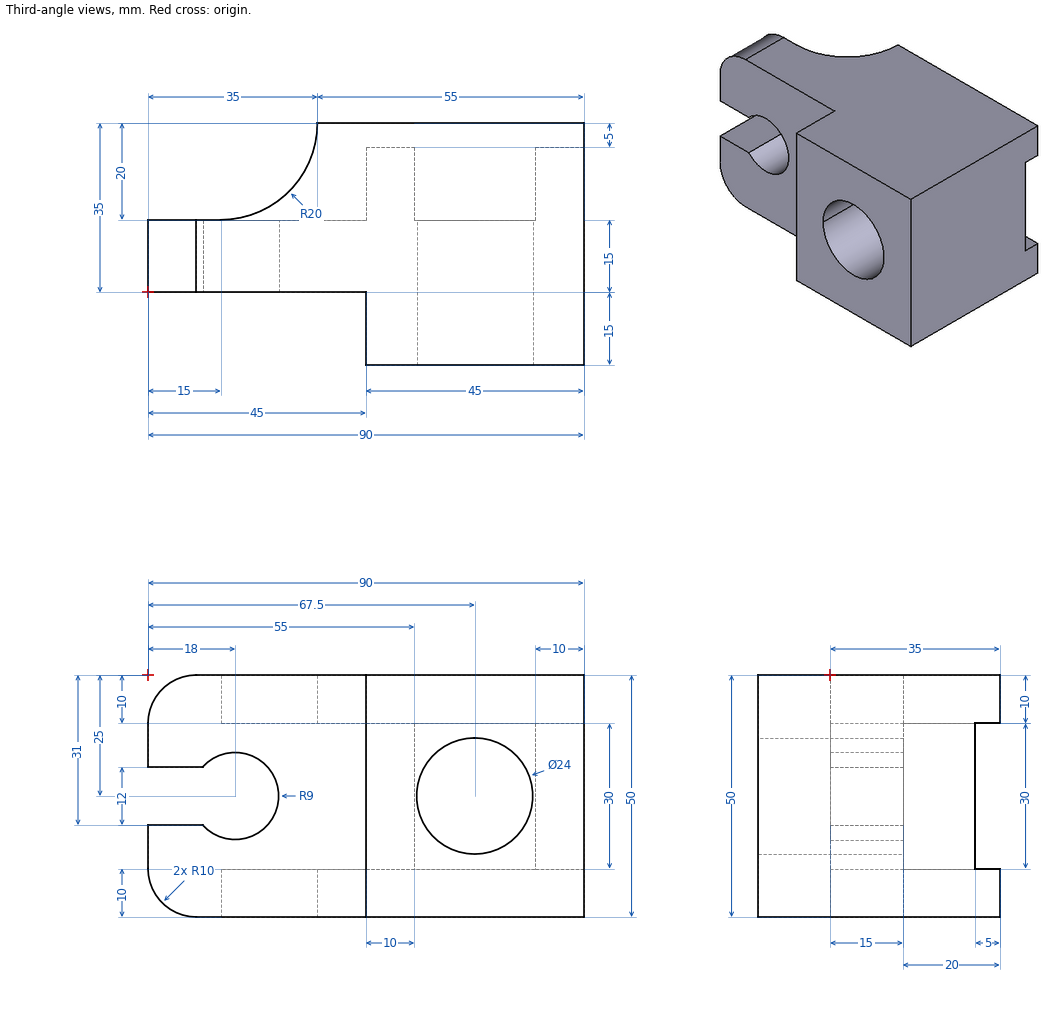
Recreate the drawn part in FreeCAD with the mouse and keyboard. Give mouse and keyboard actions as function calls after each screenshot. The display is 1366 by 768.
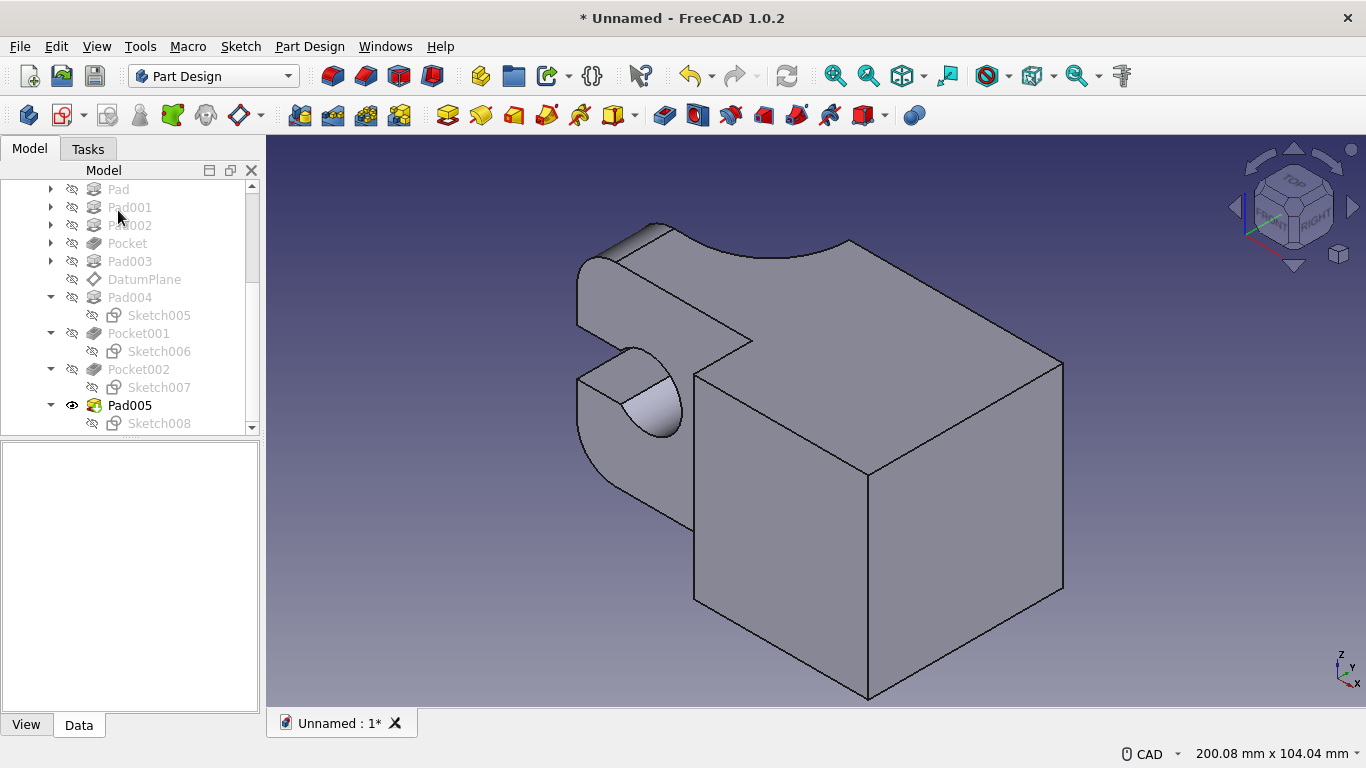
key(4)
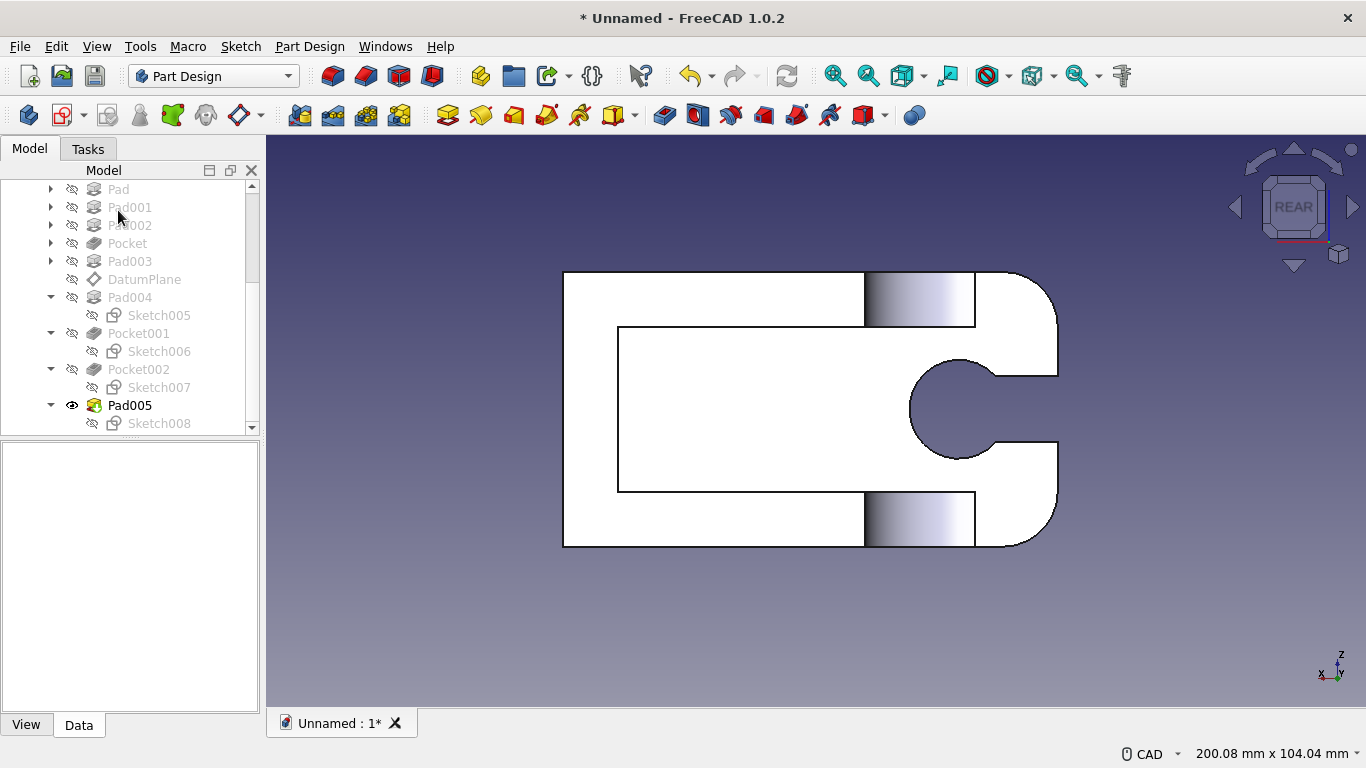
click(585, 330)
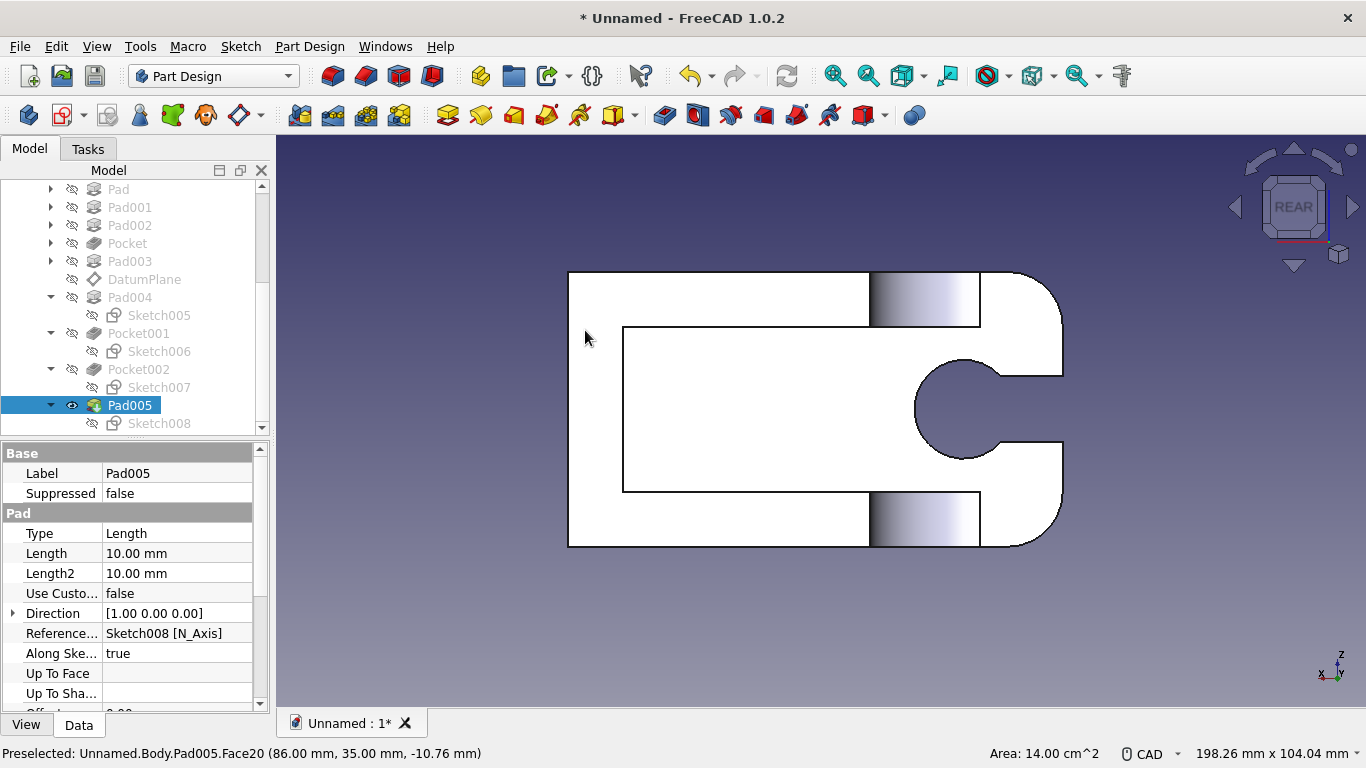
click(62, 116)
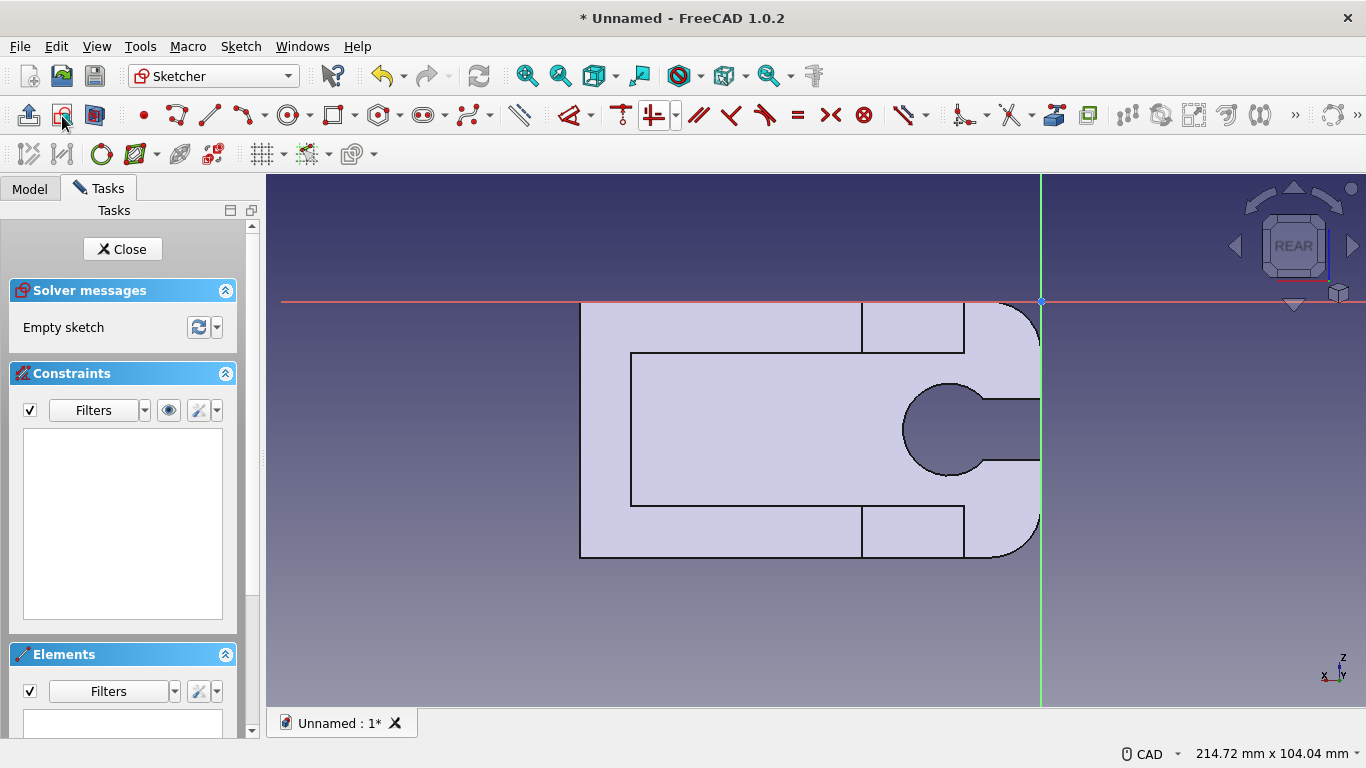
scroll(490, 421, up, 4)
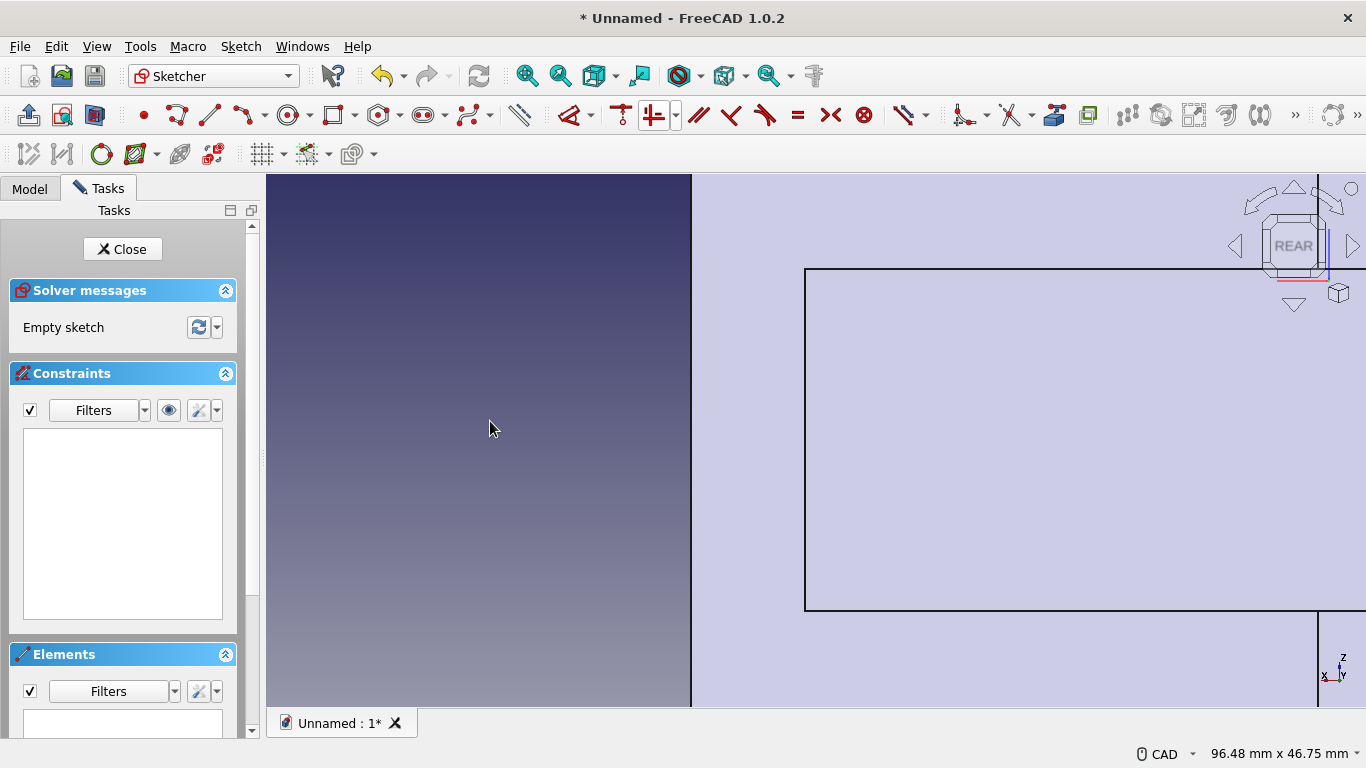
click(332, 116)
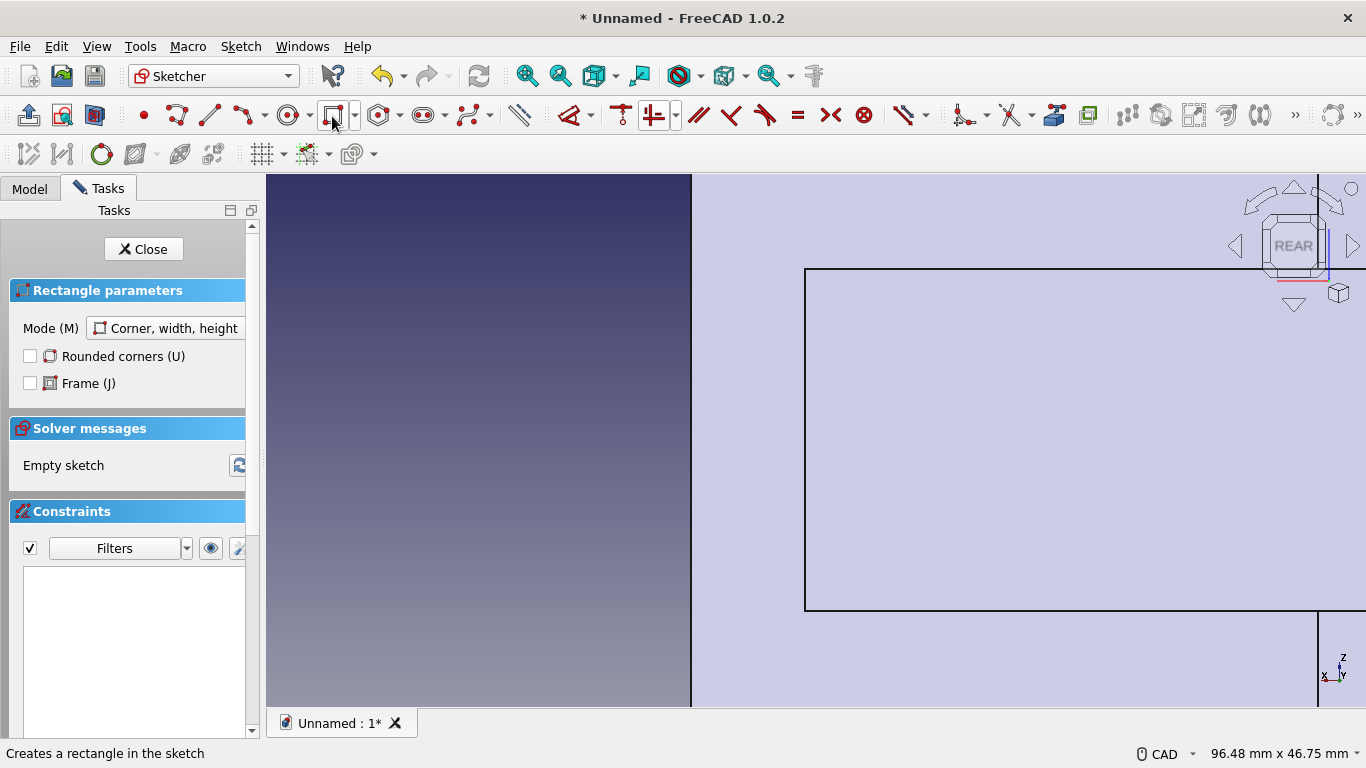
click(691, 269)
click(805, 611)
key(Escape)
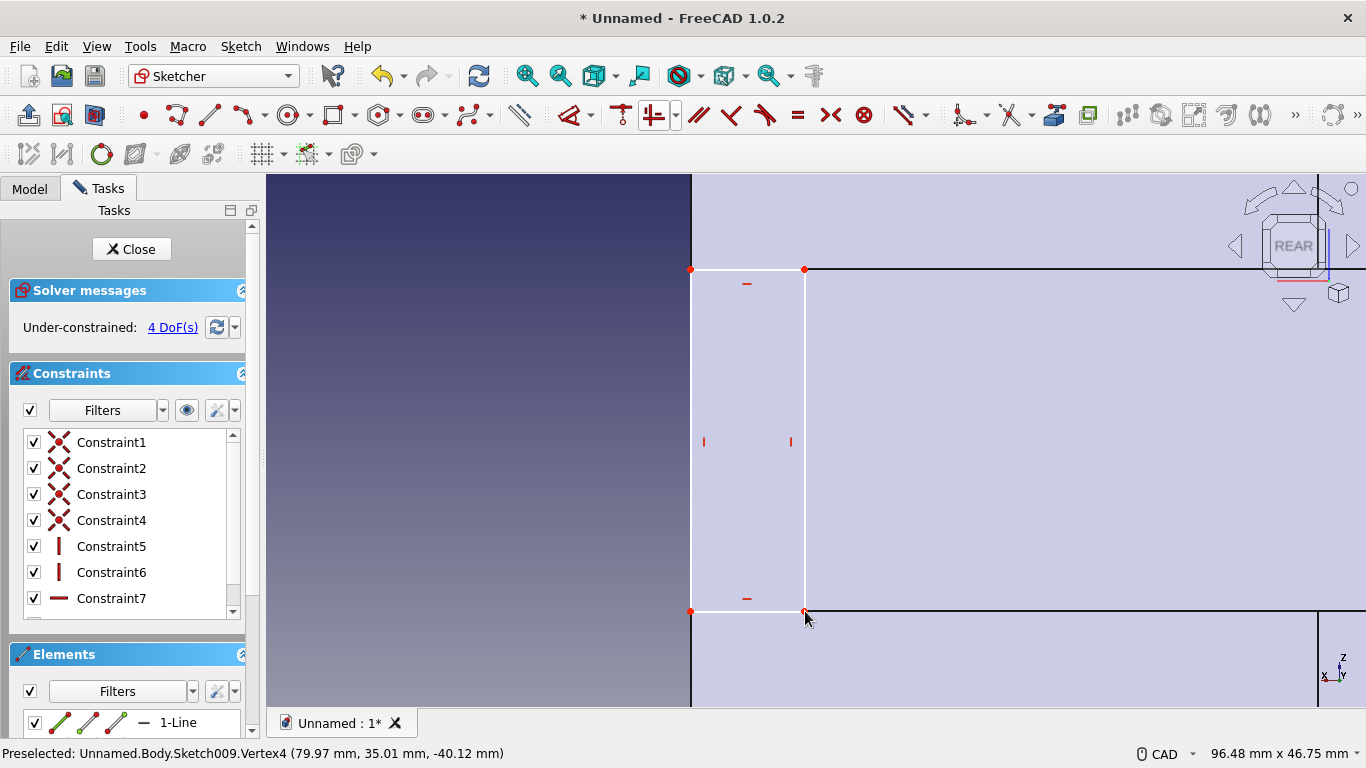
key(d)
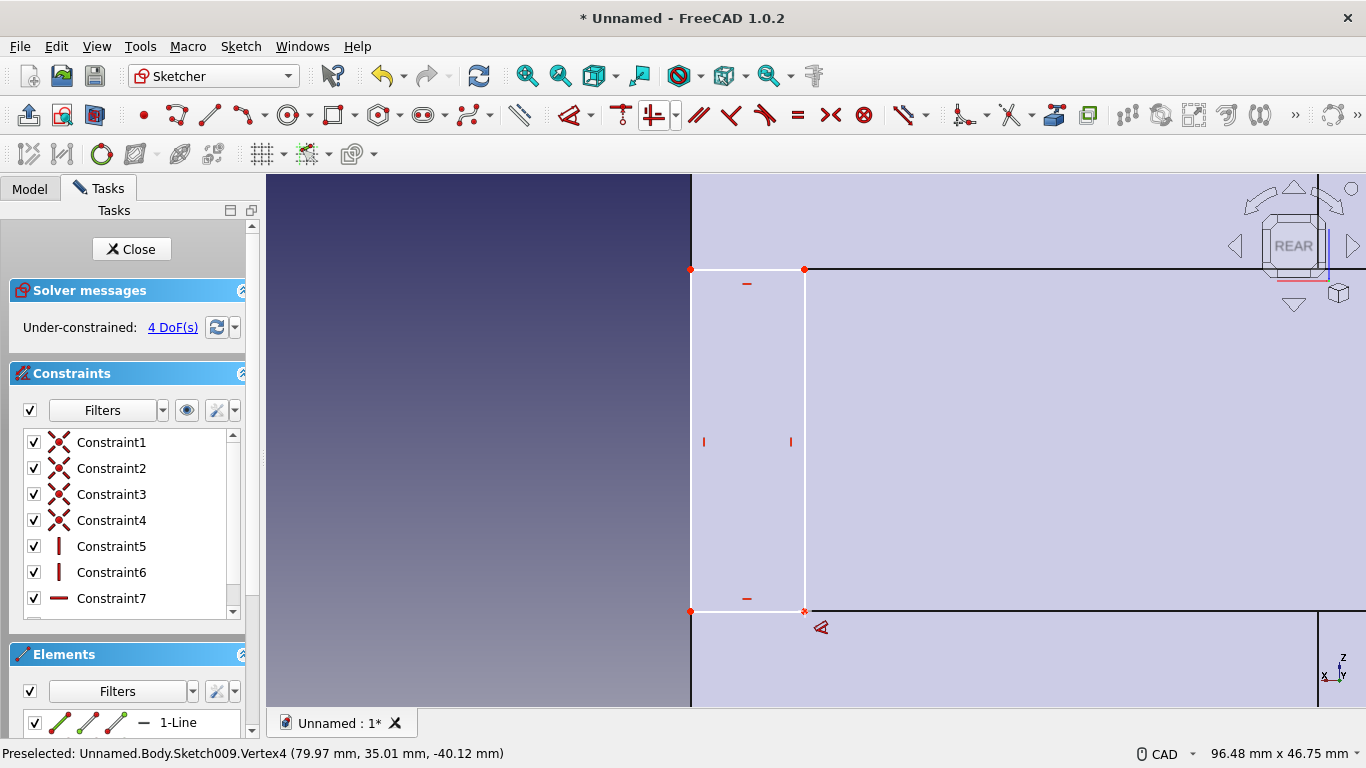
click(691, 373)
click(657, 441)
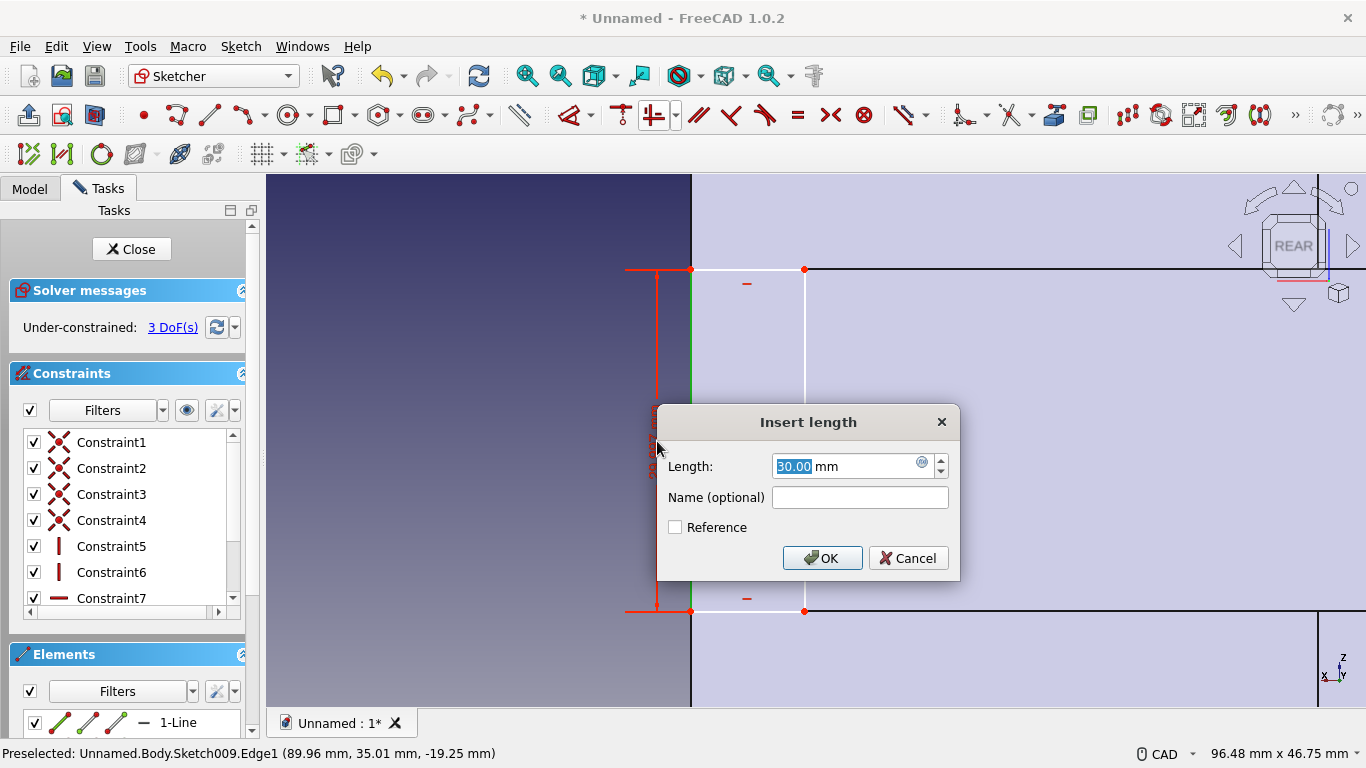
text(30)
key(Return)